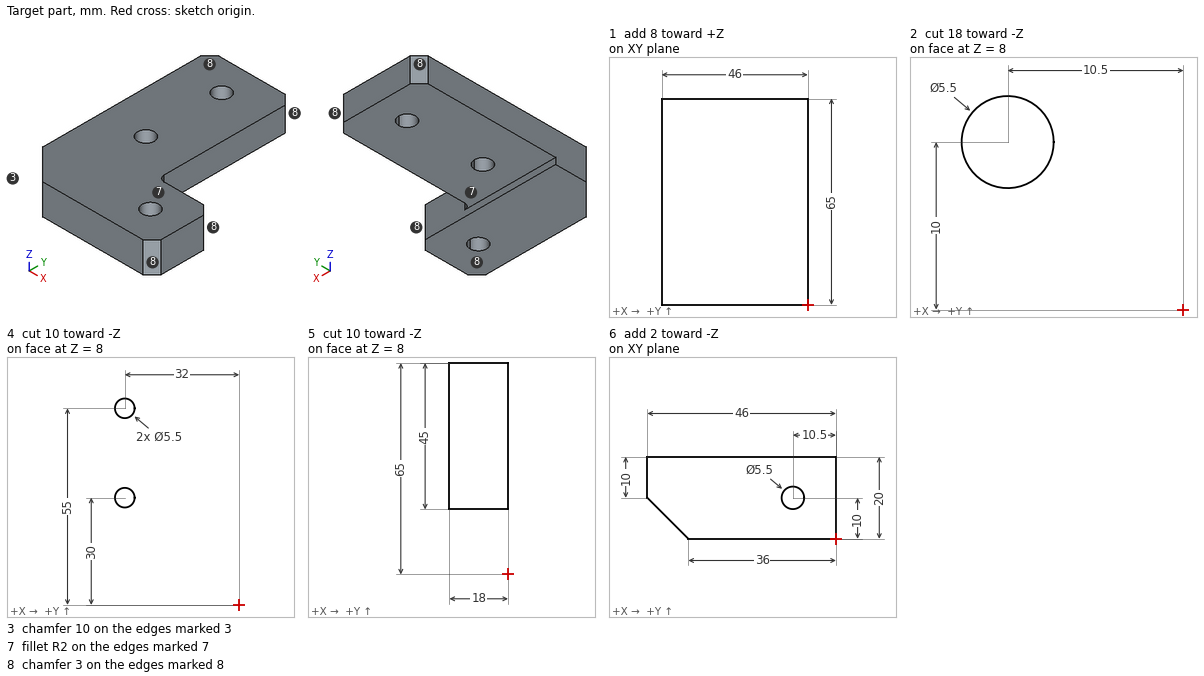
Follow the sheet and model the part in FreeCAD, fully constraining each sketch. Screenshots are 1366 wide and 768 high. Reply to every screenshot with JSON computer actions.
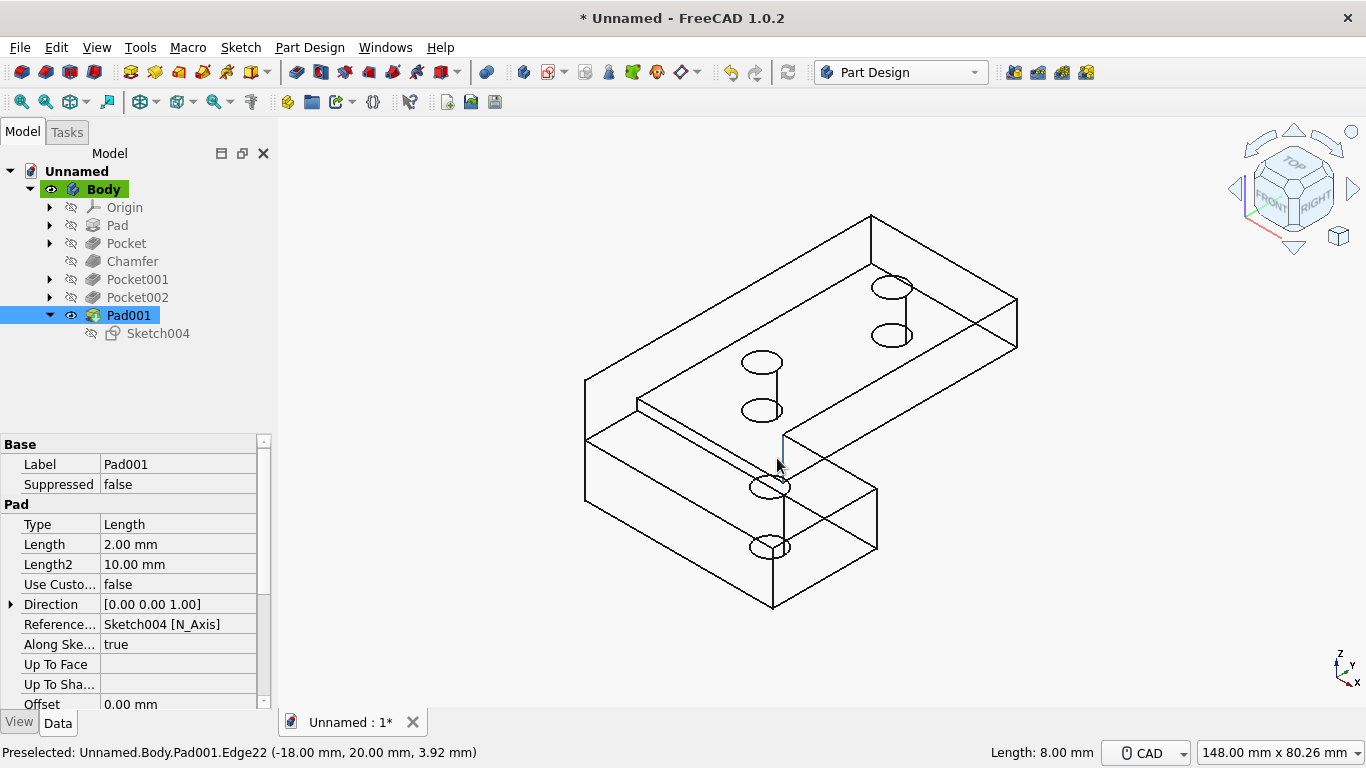
{"action": "key", "text": "v 1"}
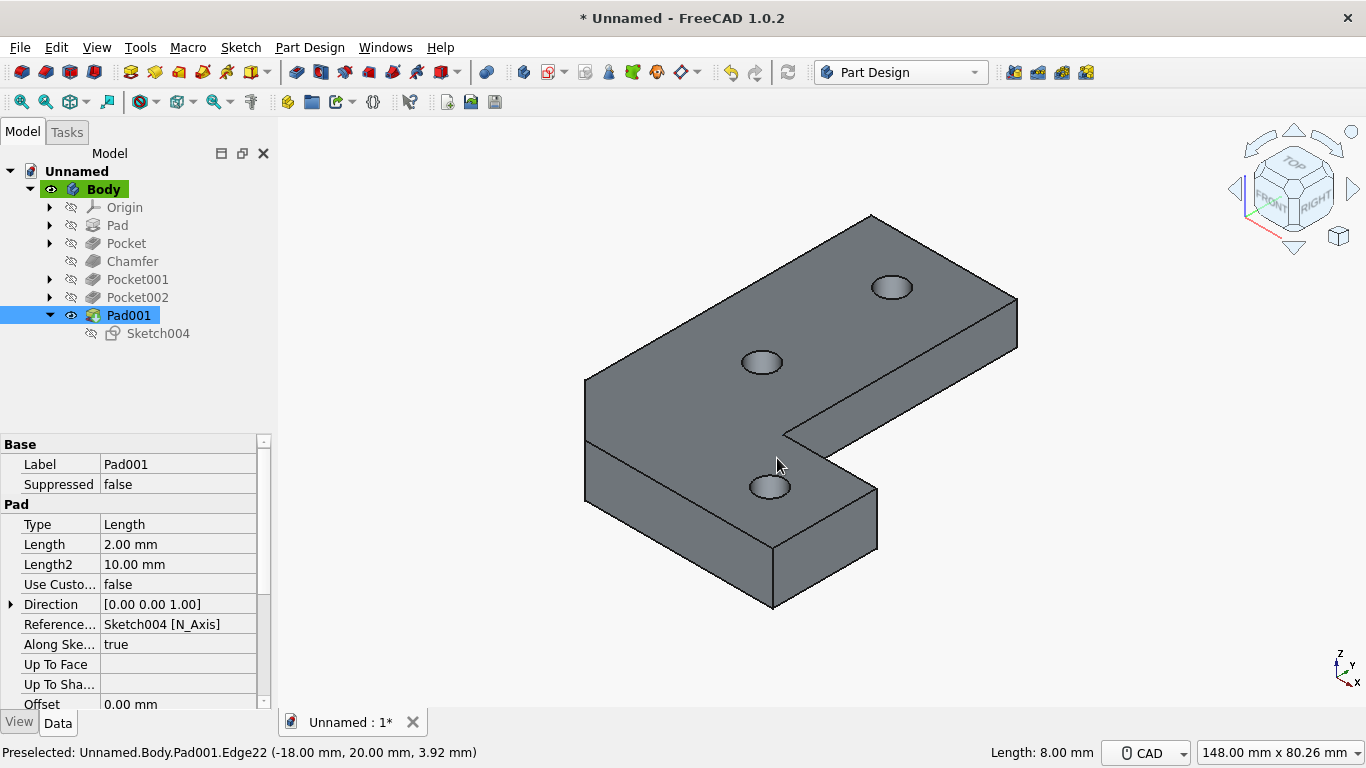
{"action": "left_click", "coordinate": [22, 72]}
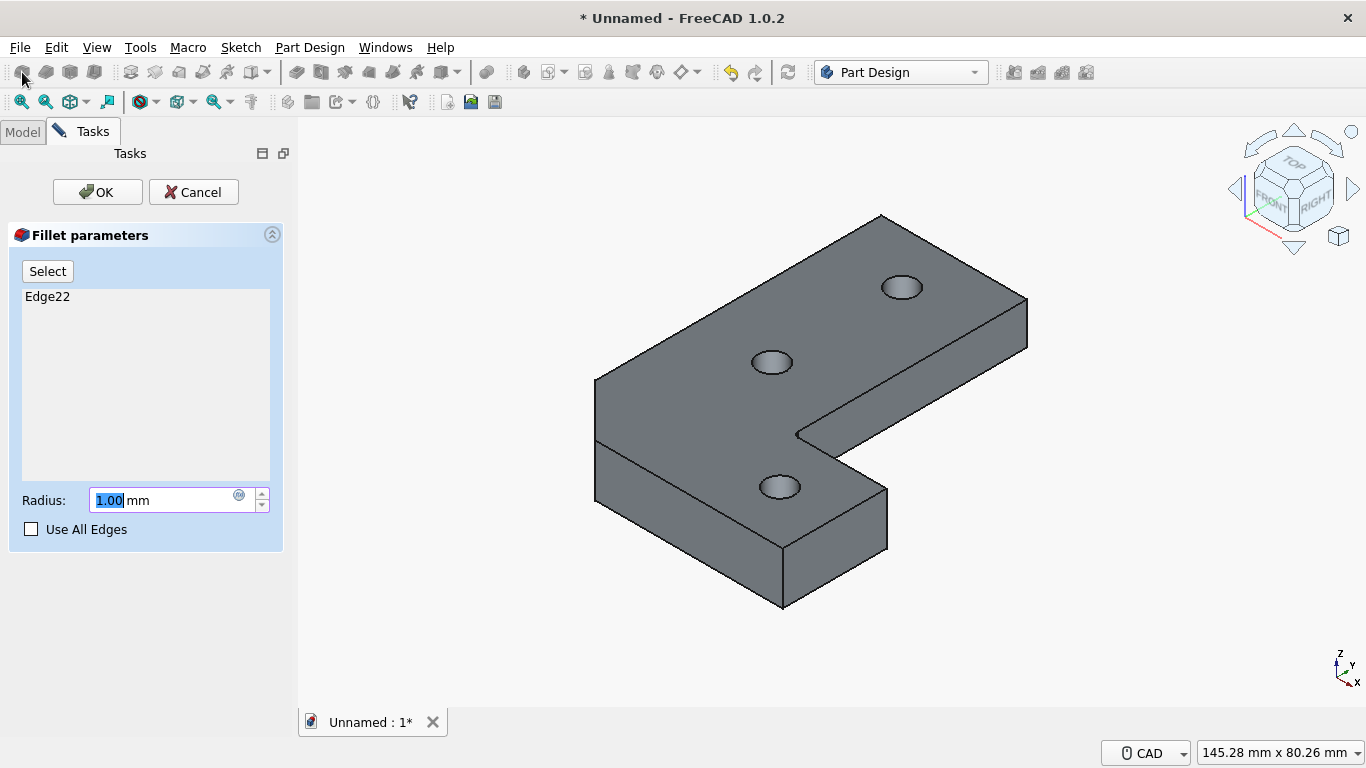
{"action": "type", "text": "2"}
{"action": "key", "text": "Tab"}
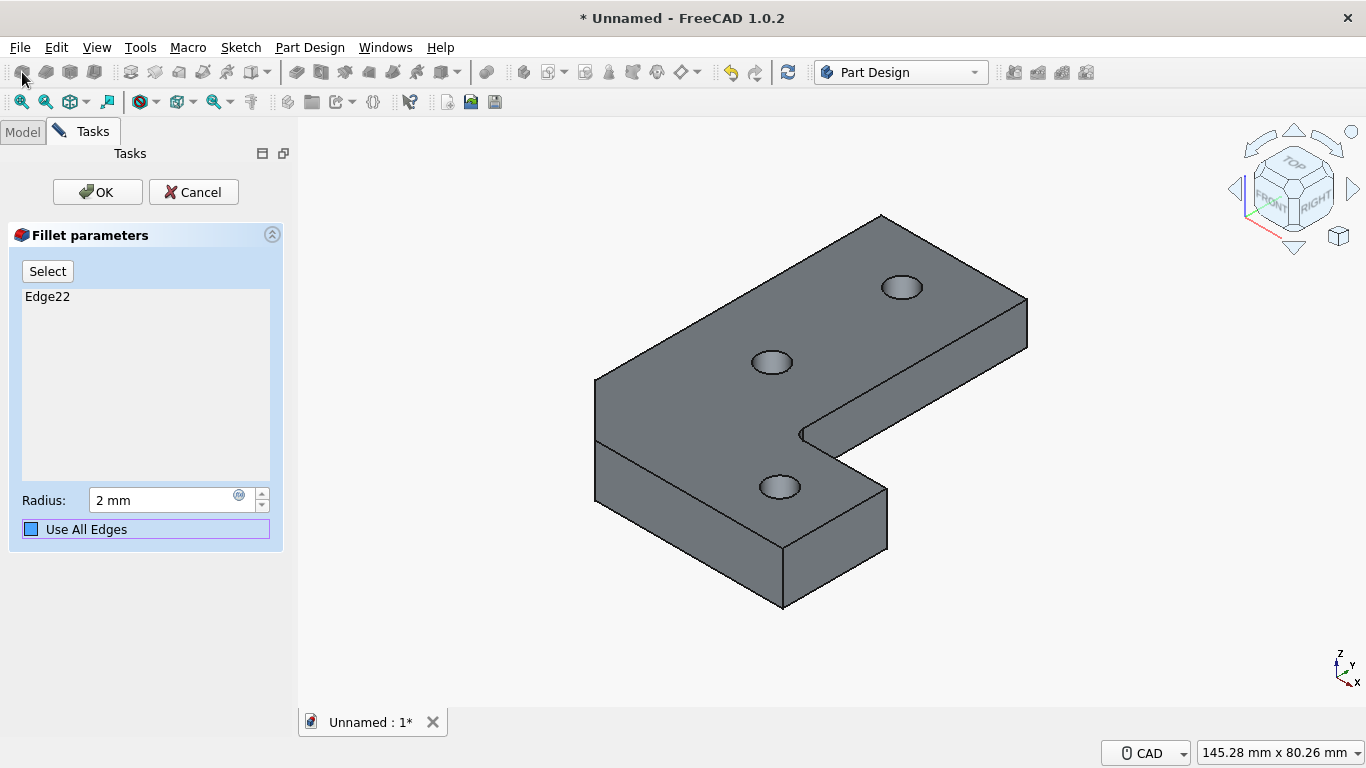
{"action": "left_click", "coordinate": [98, 192]}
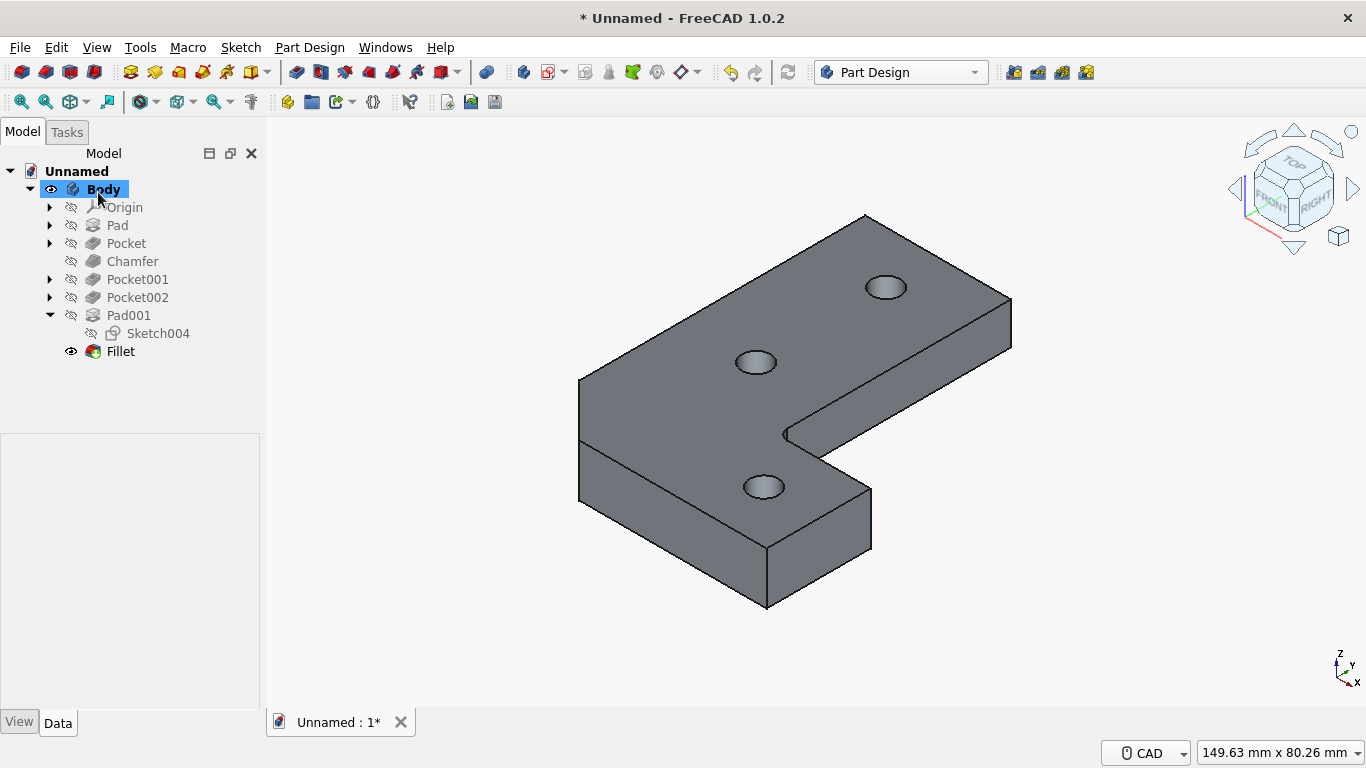
{"action": "left_click", "coordinate": [767, 578]}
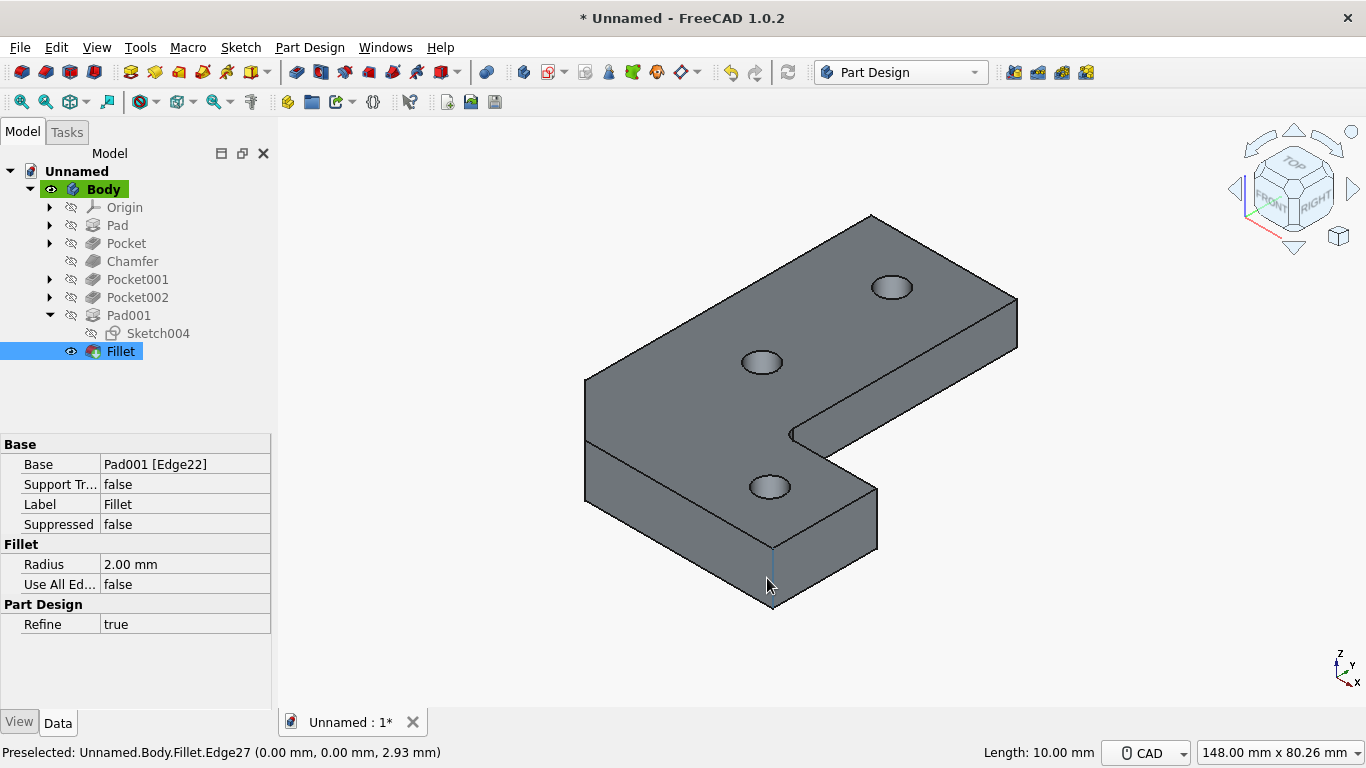
{"action": "key", "text": "2"}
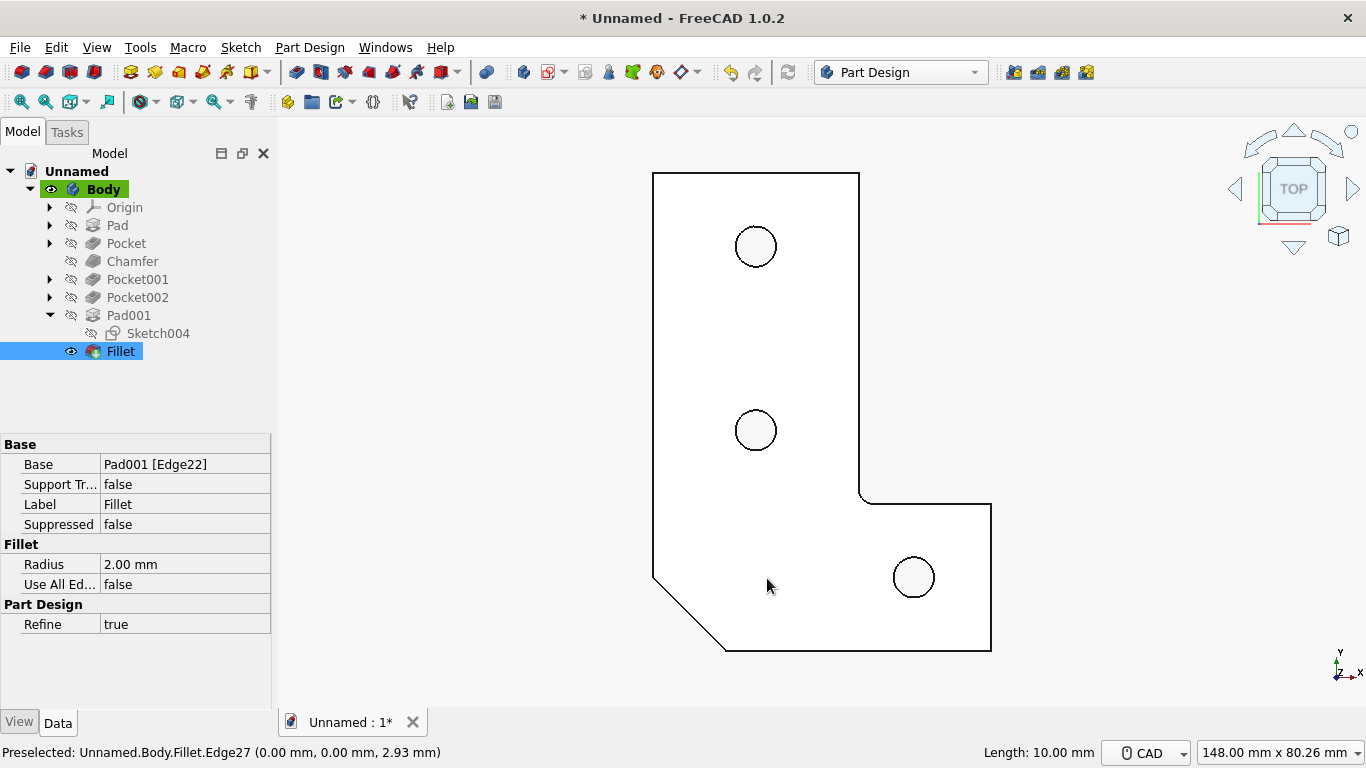
{"action": "key", "text": "0"}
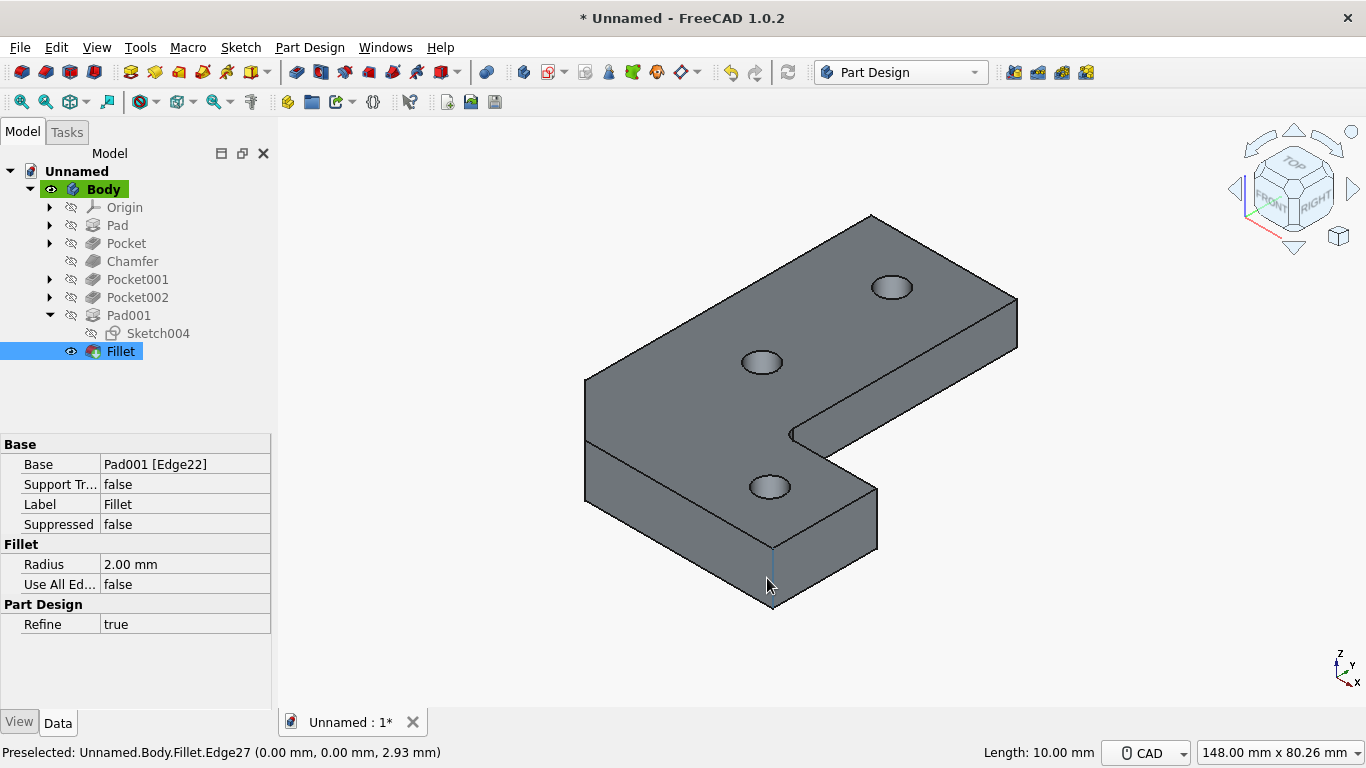
{"action": "key", "text": "1"}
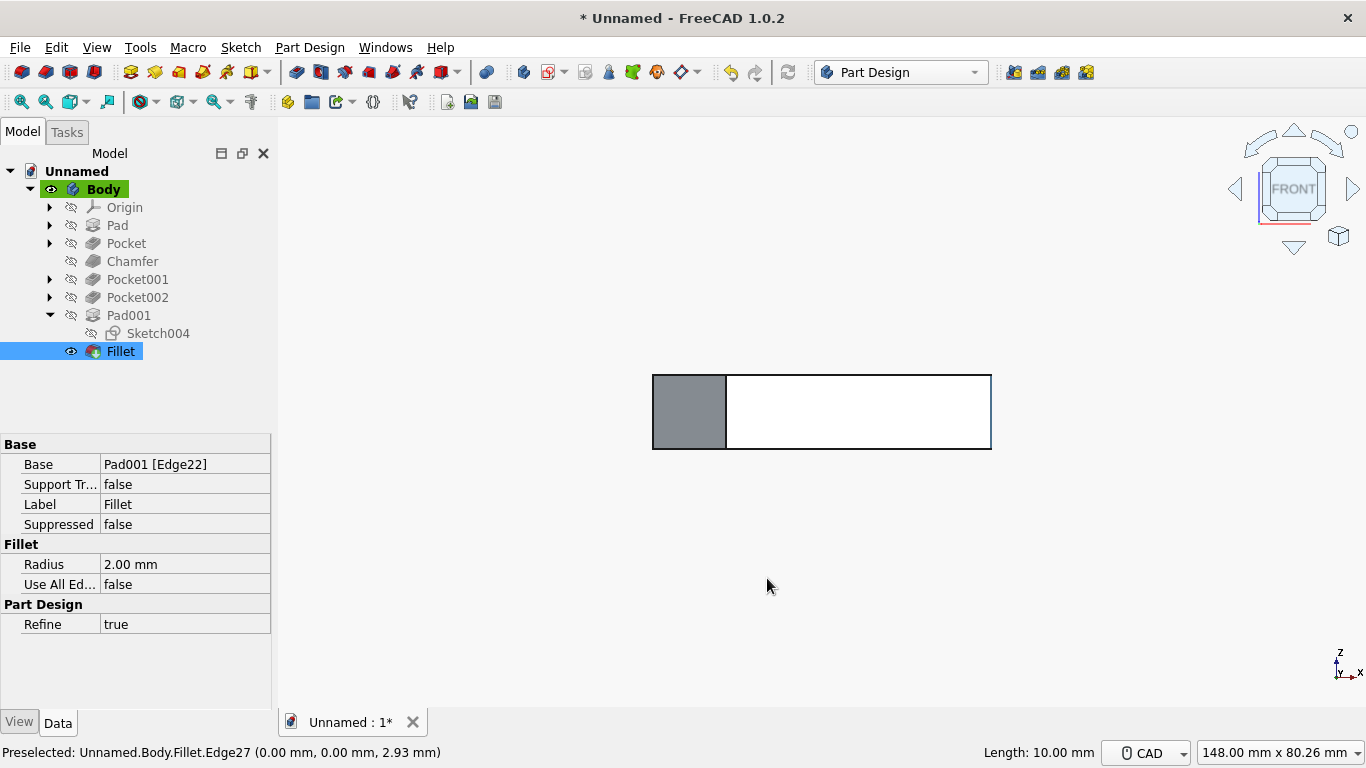
{"action": "left_click", "coordinate": [22, 102]}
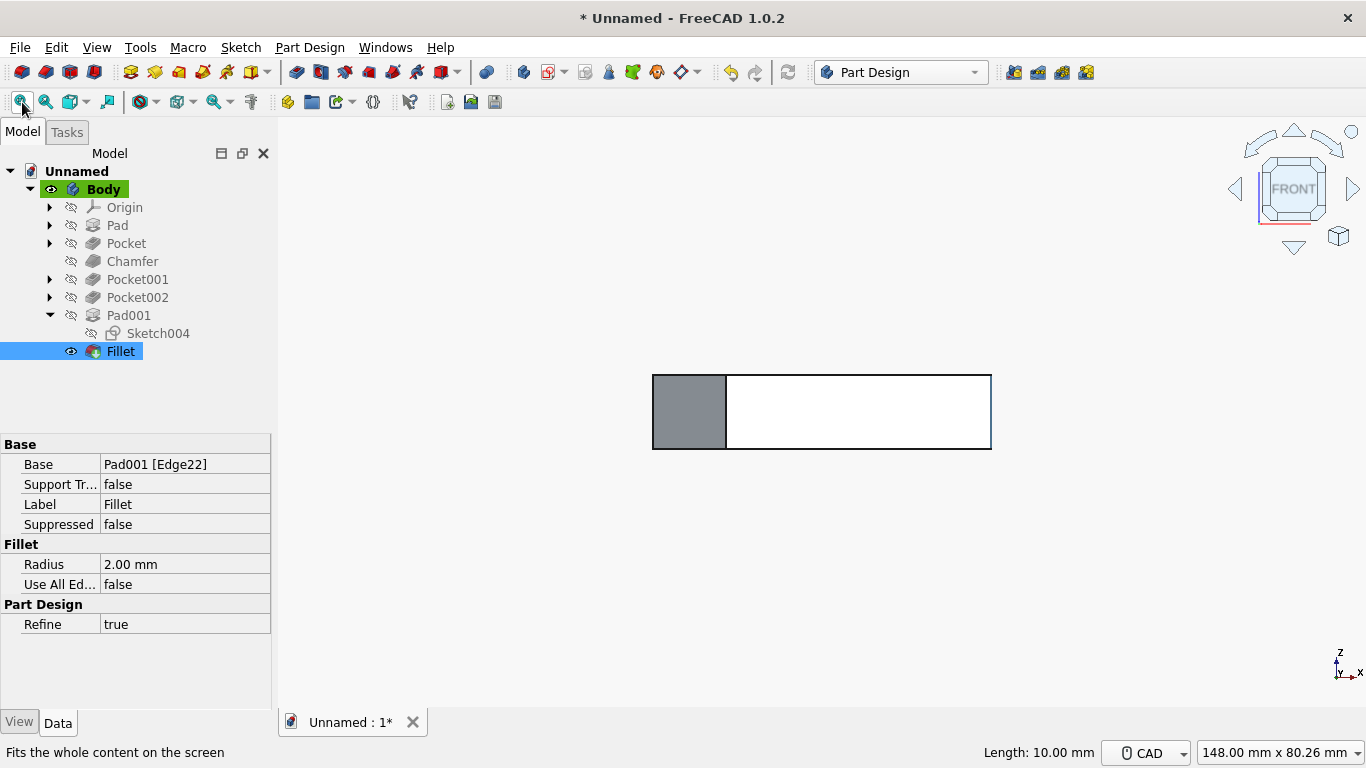
{"action": "key", "text": "3"}